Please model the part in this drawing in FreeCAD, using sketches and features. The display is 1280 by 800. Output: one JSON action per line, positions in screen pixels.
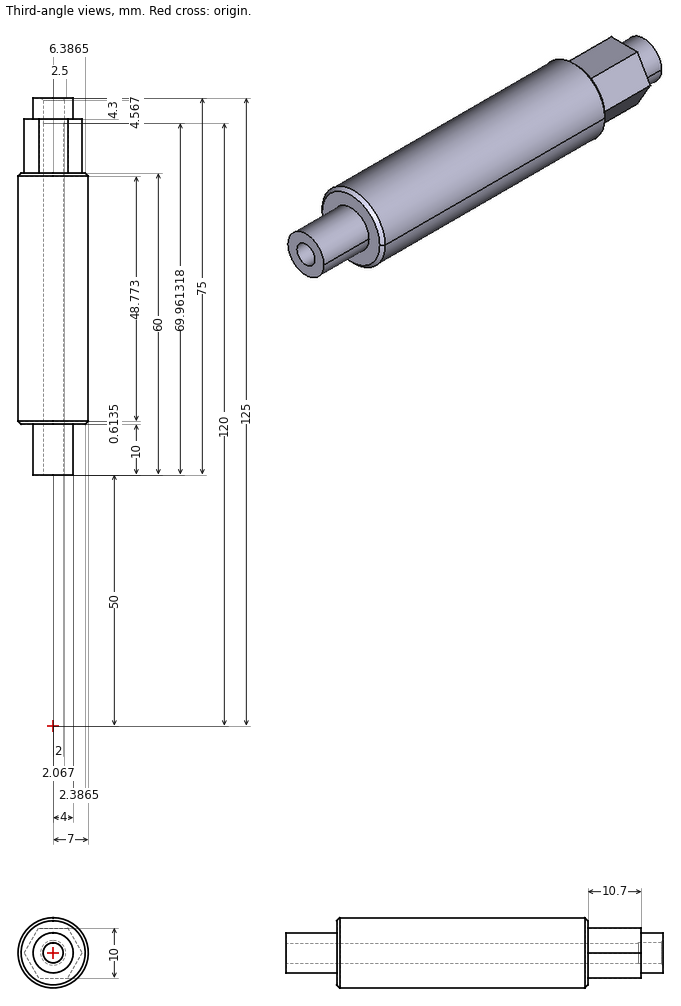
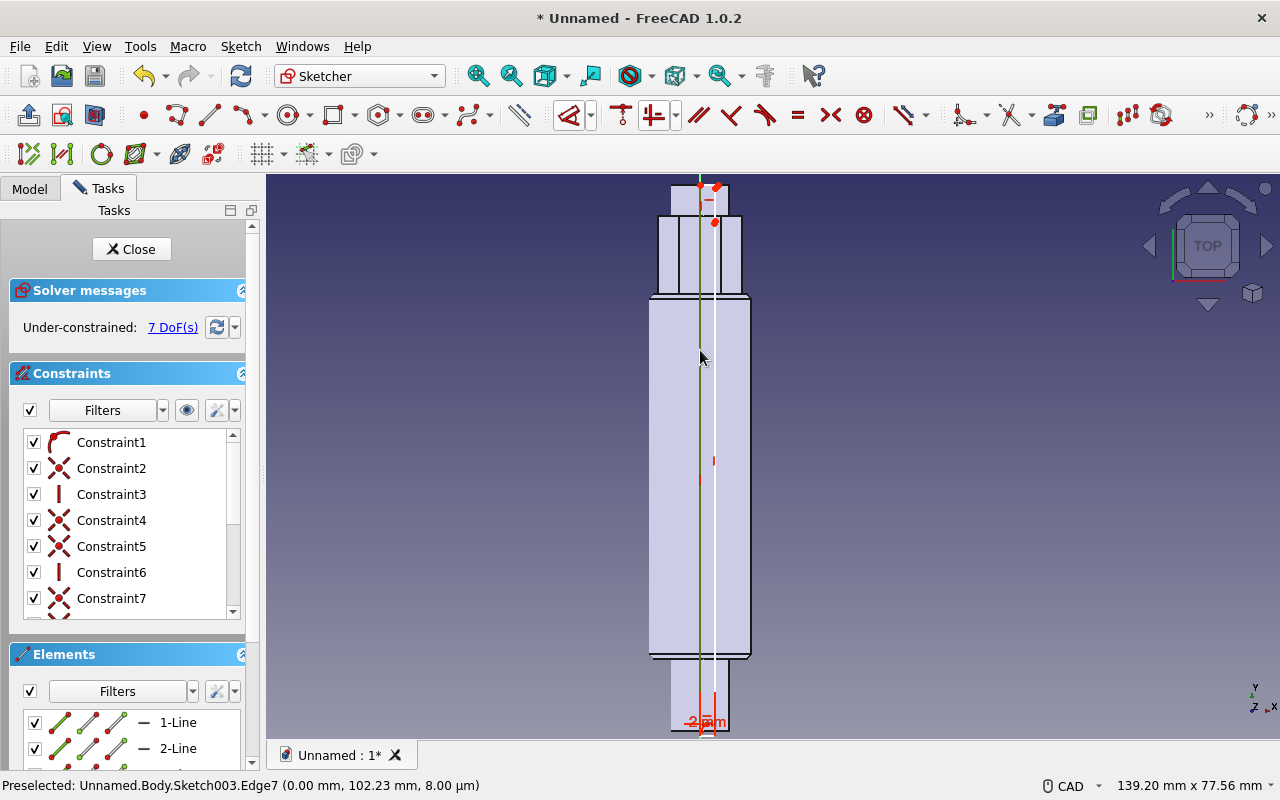
{"action": "key", "text": "i"}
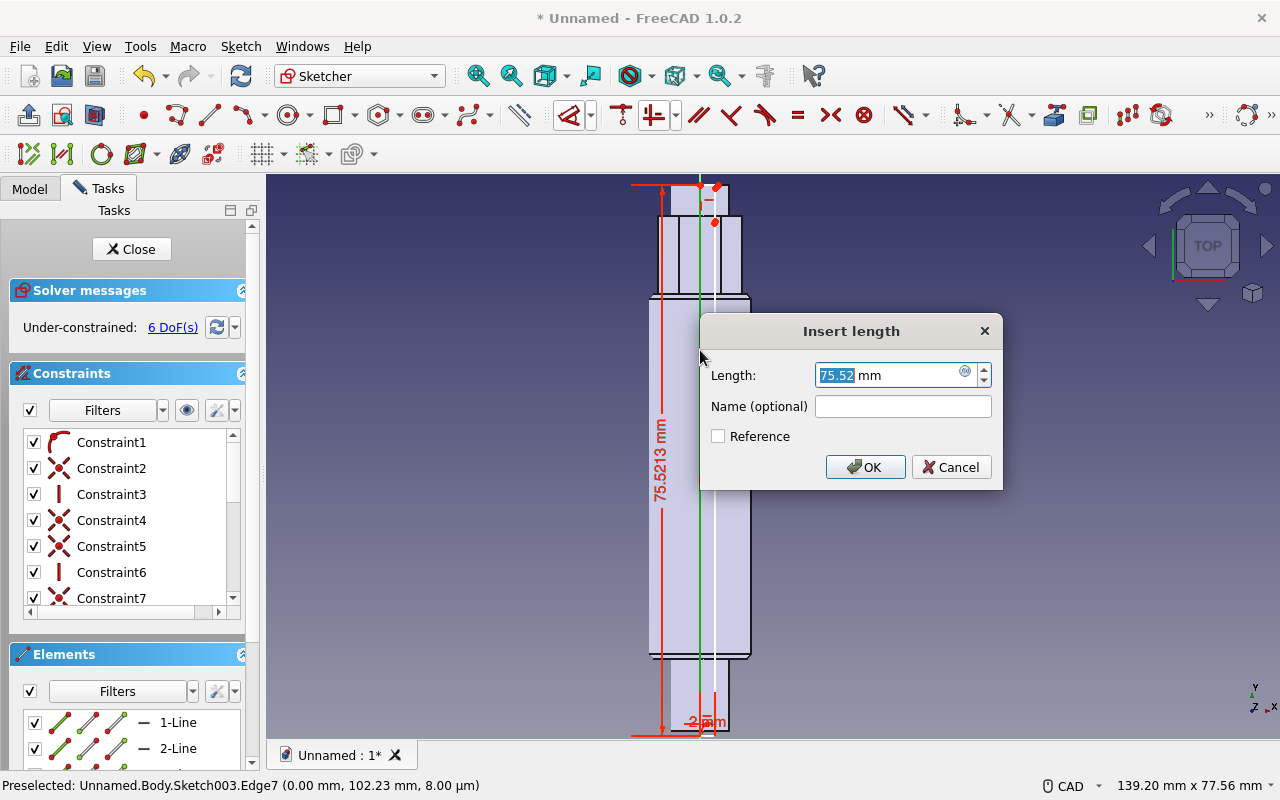
{"action": "type", "text": "75"}
{"action": "key", "text": "Return"}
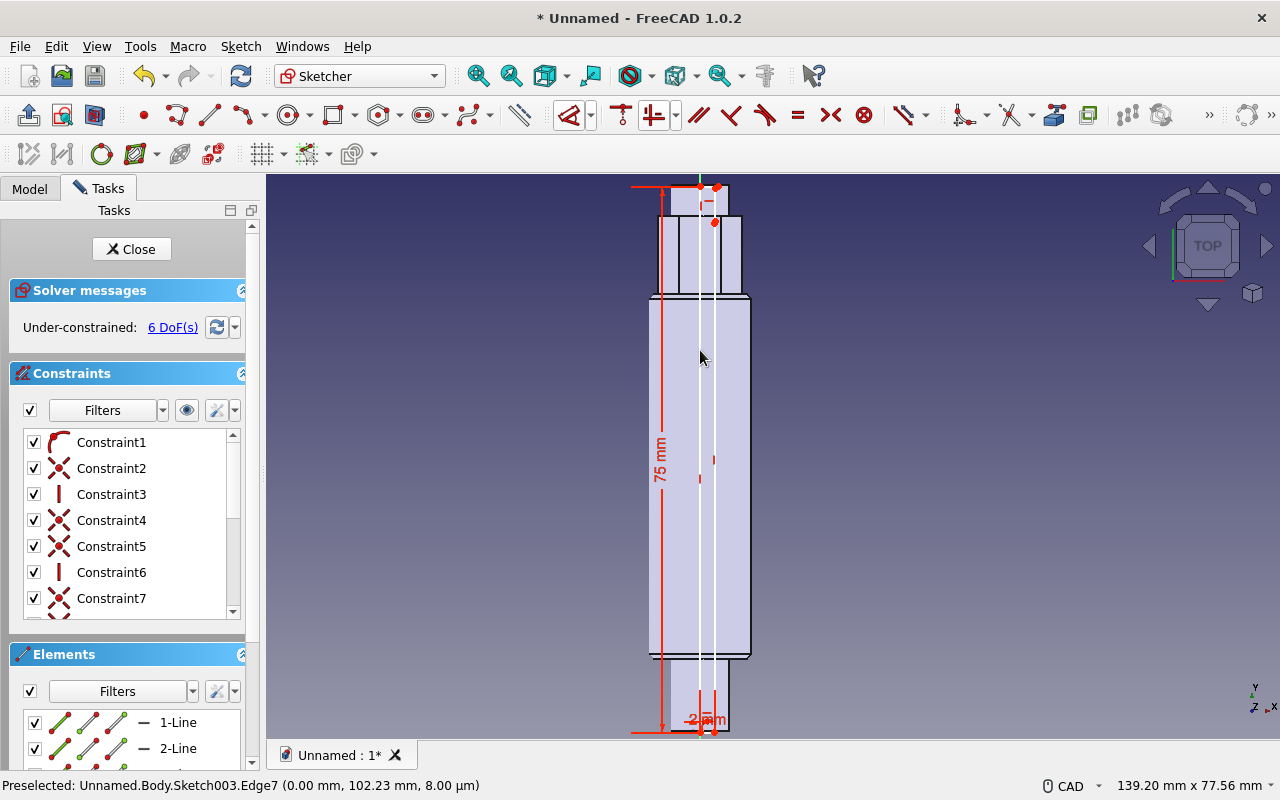
{"action": "scroll", "coordinate": [702, 349], "scroll_direction": "down", "scroll_amount": 5}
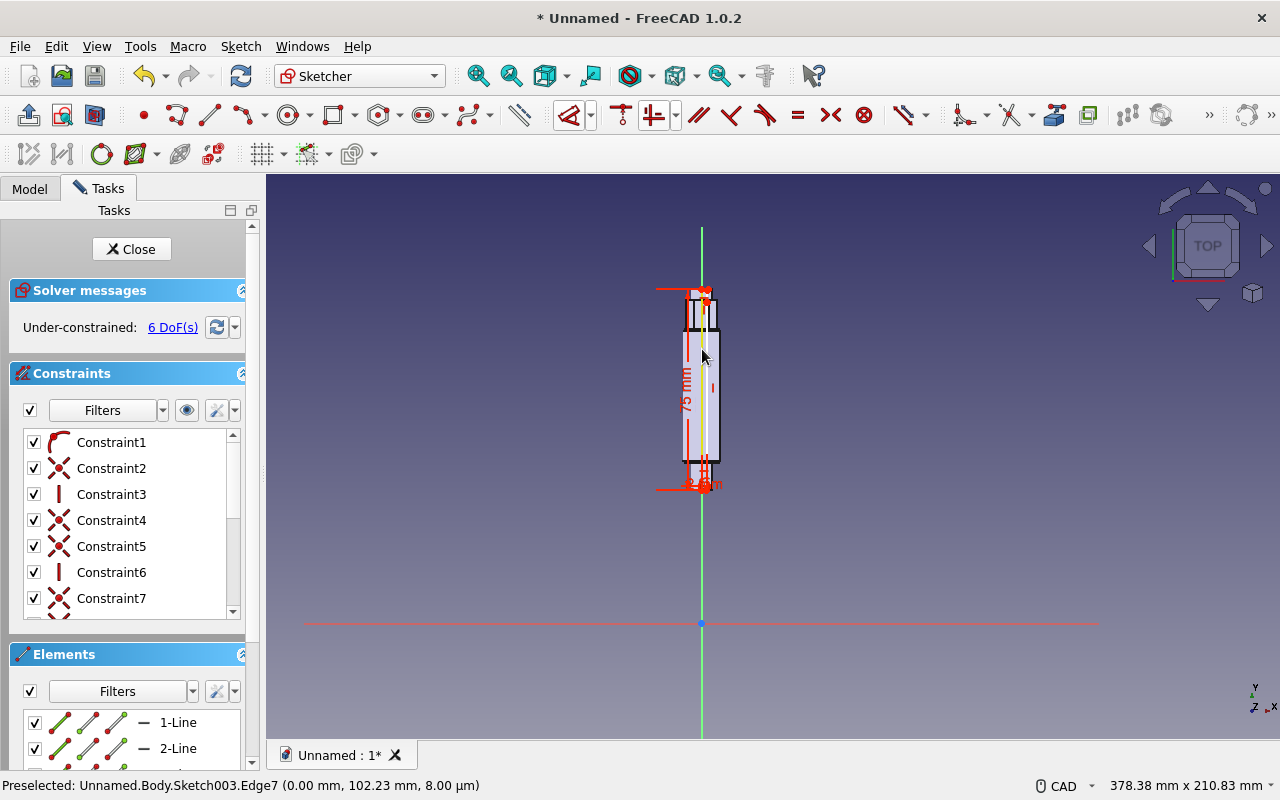
{"action": "scroll", "coordinate": [704, 289], "scroll_direction": "up", "scroll_amount": 9}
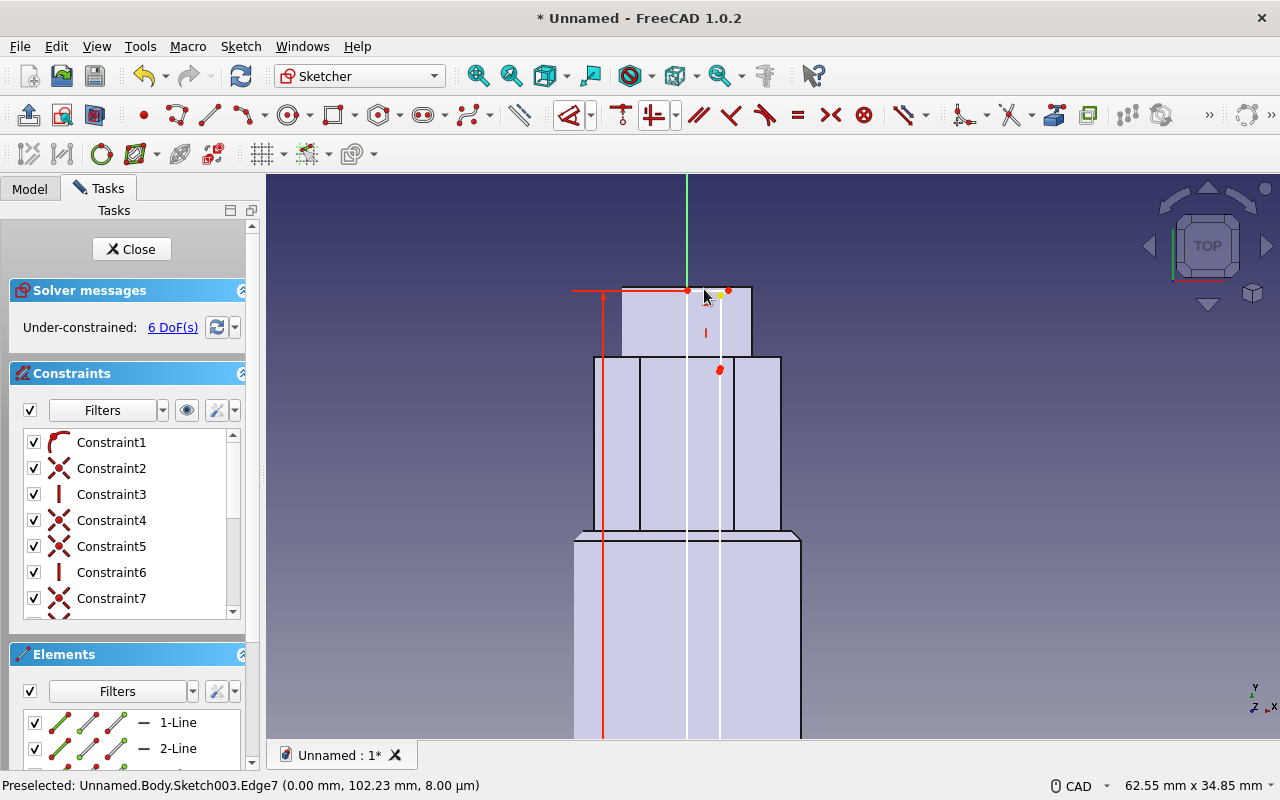
{"action": "left_click", "coordinate": [704, 291]}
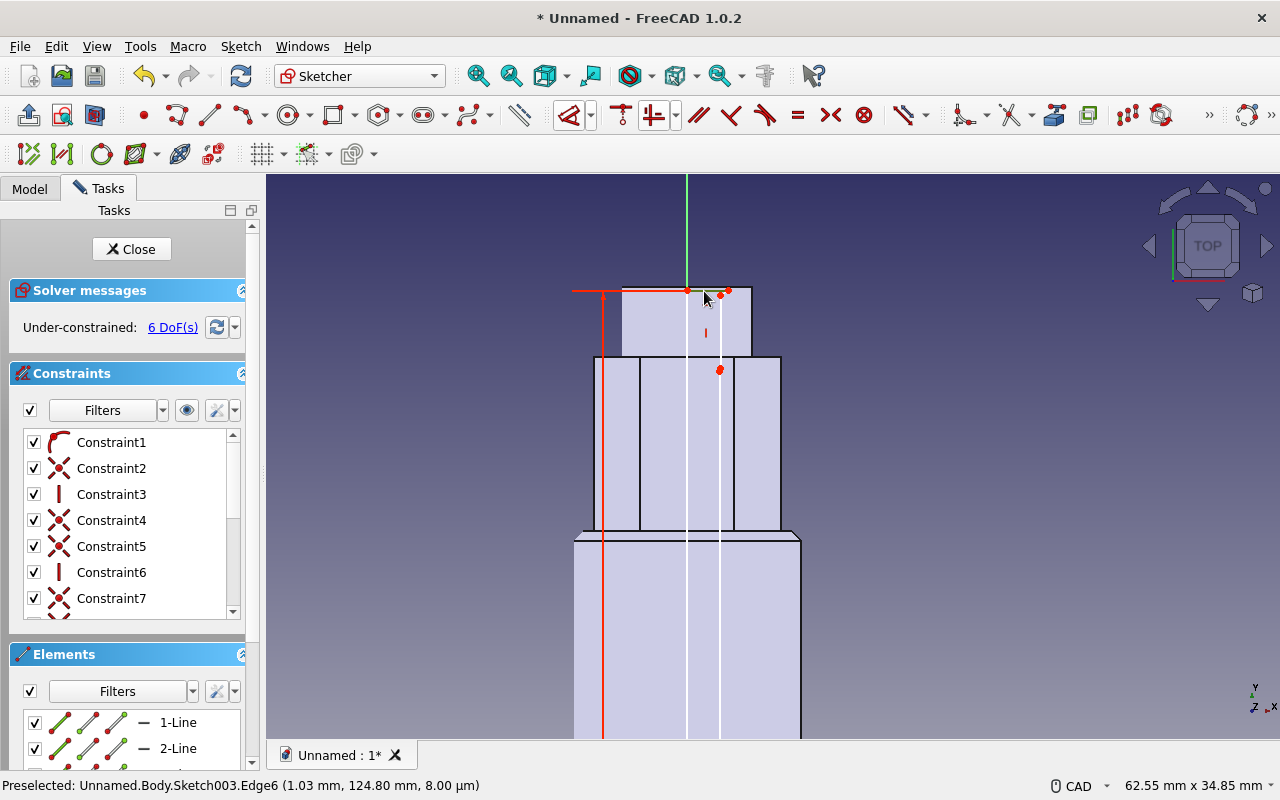
{"action": "left_click", "coordinate": [590, 116]}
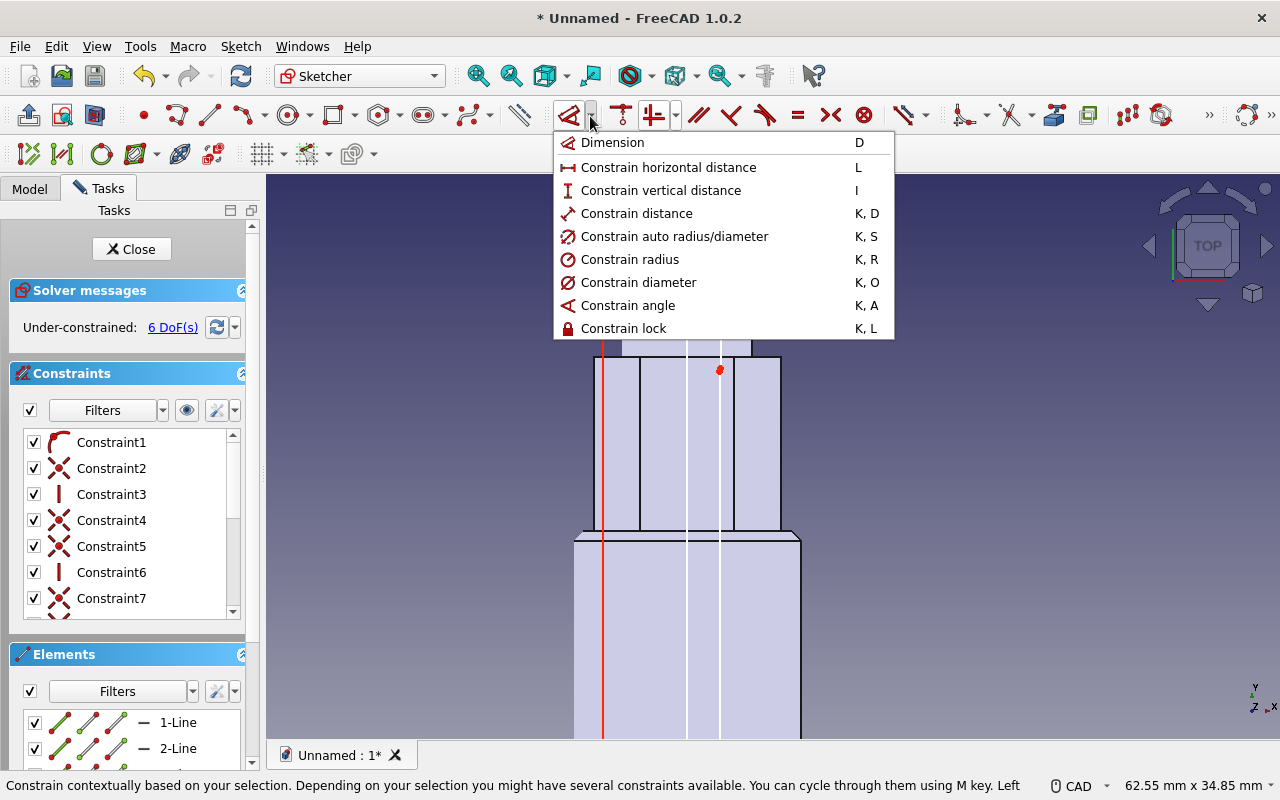
{"action": "left_click", "coordinate": [724, 168]}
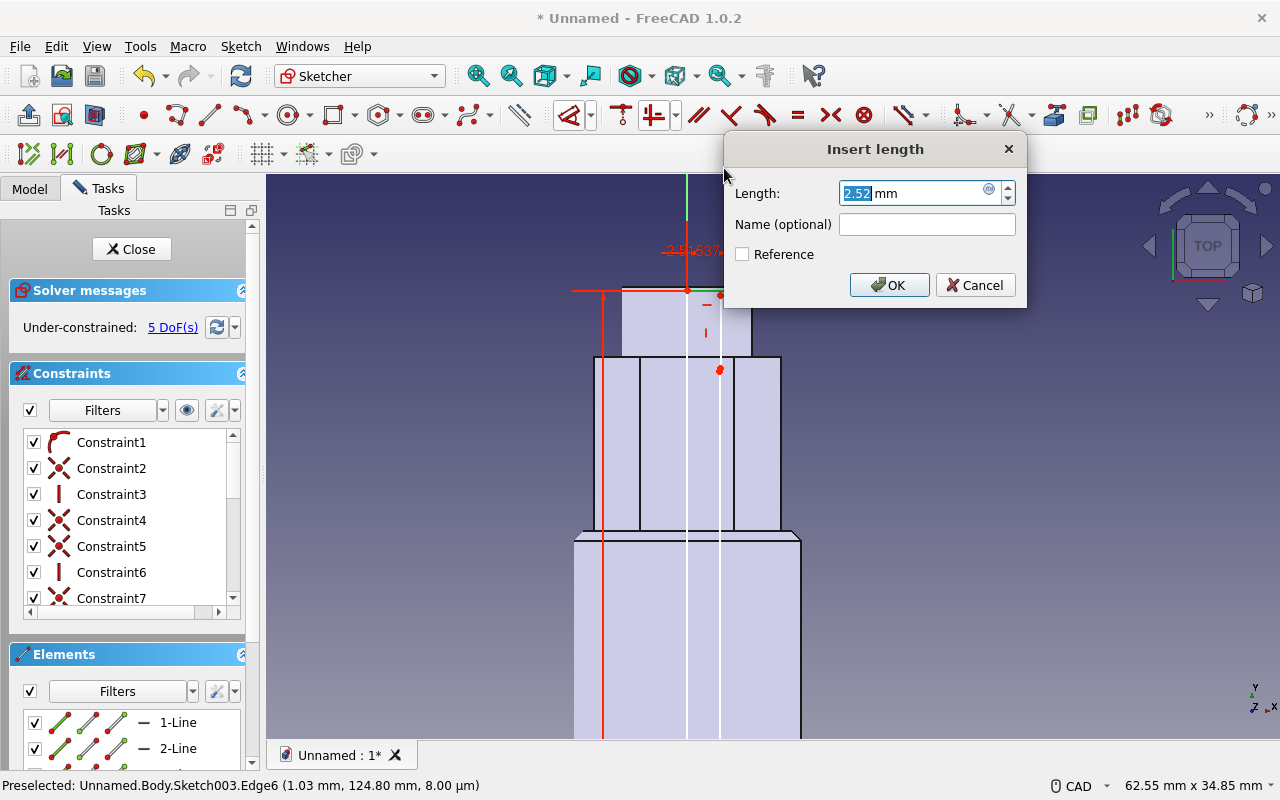
{"action": "type", "text": "2.5"}
{"action": "key", "text": "Return"}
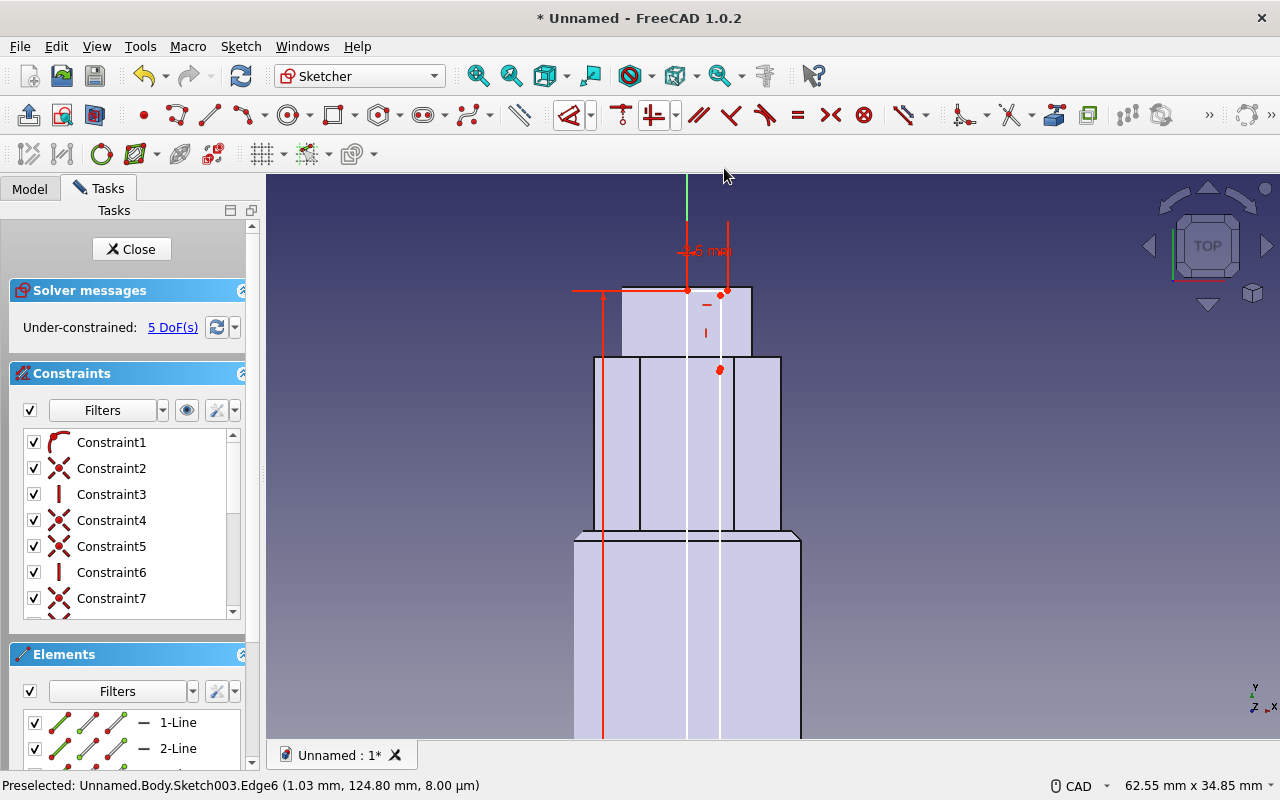
{"action": "scroll", "coordinate": [704, 289], "scroll_direction": "down", "scroll_amount": 9}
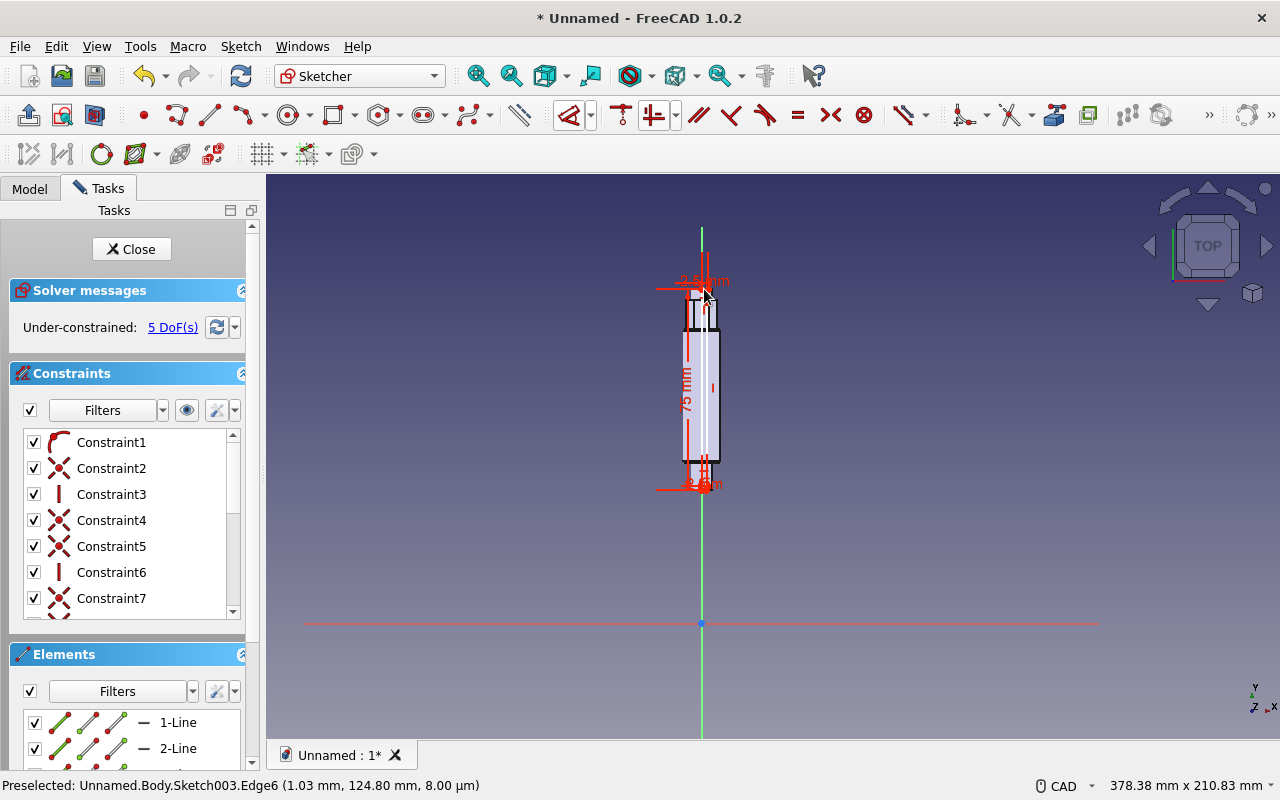
{"action": "scroll", "coordinate": [702, 490], "scroll_direction": "up", "scroll_amount": 5}